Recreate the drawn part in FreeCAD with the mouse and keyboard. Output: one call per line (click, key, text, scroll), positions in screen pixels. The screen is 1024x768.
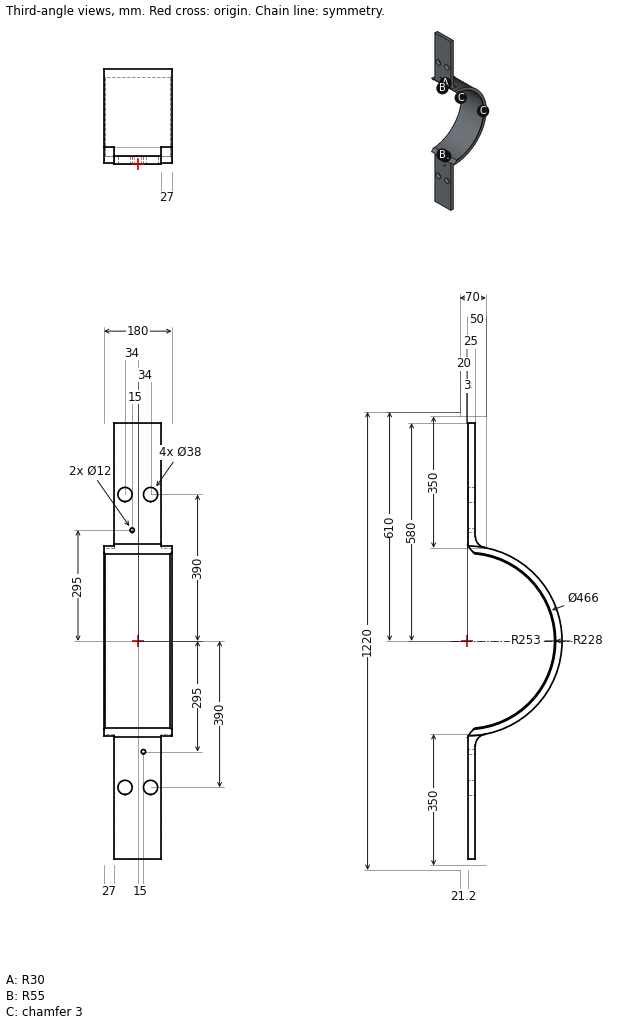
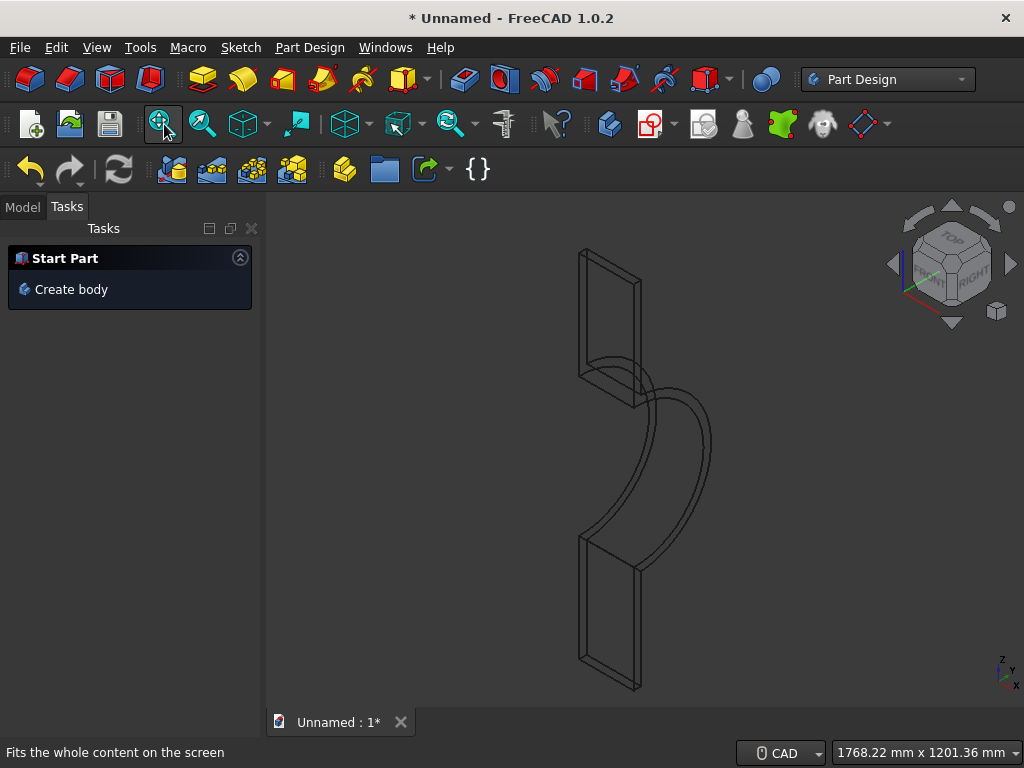
click(614, 378)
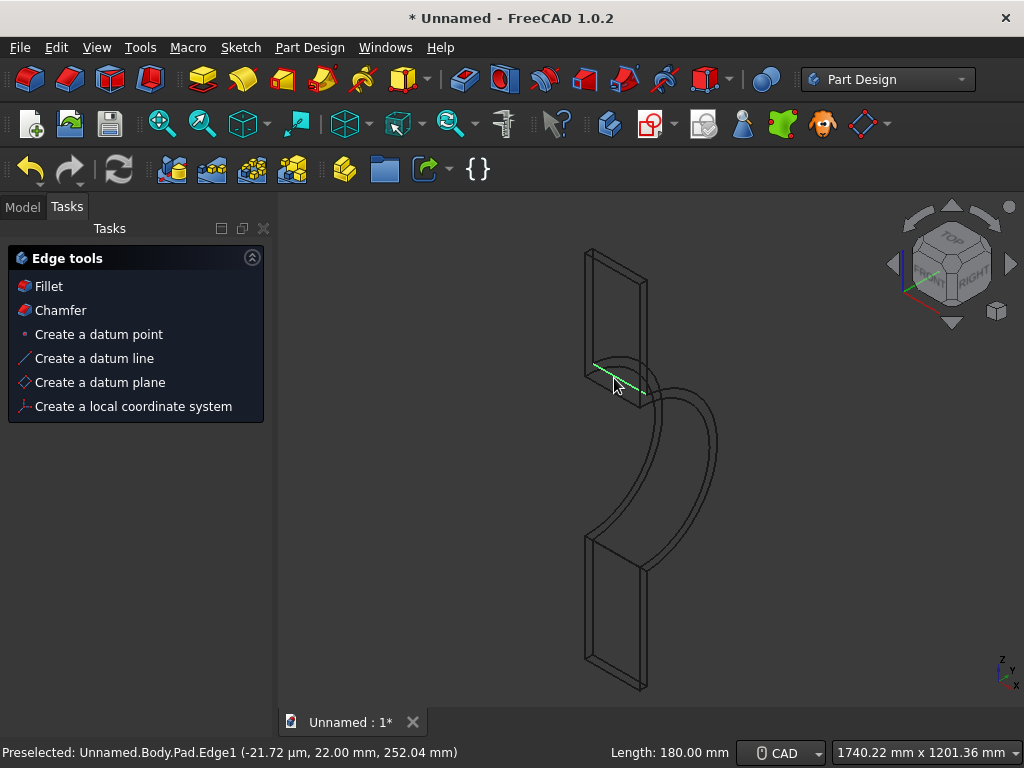
key(2)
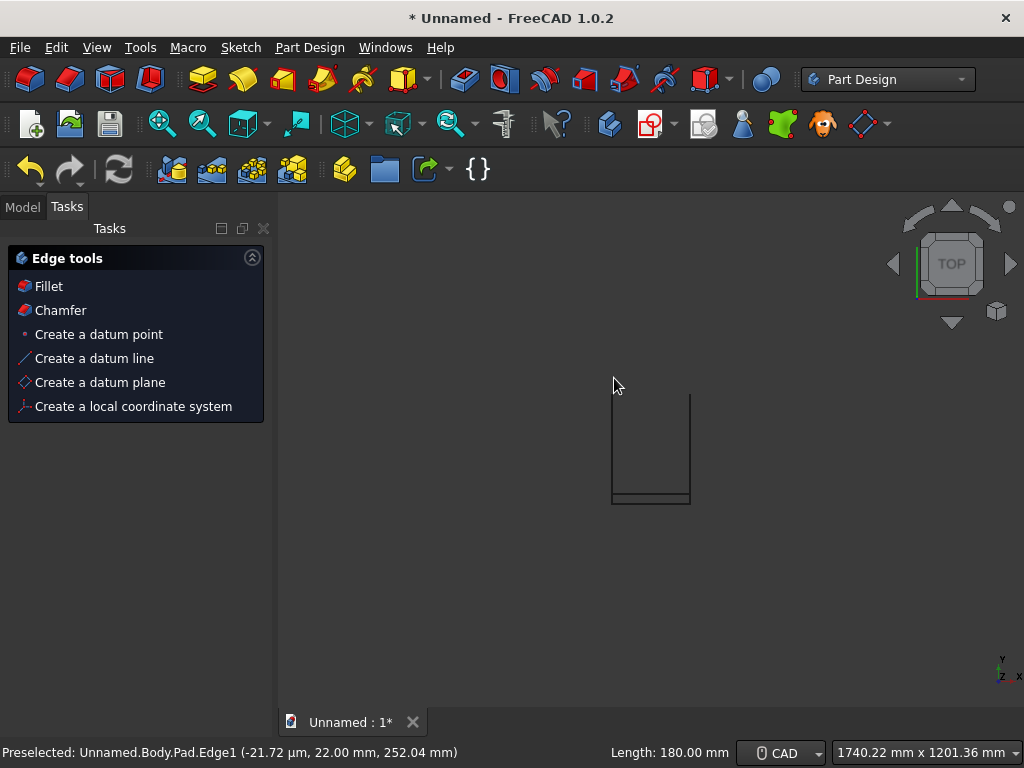
click(164, 124)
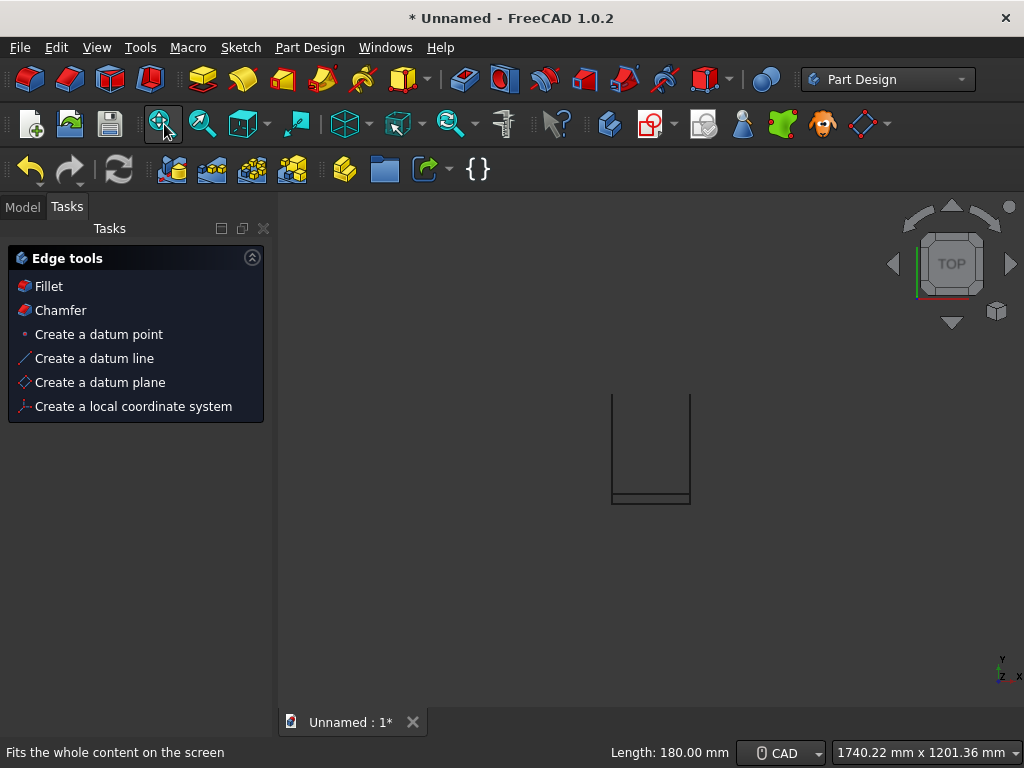
key(1)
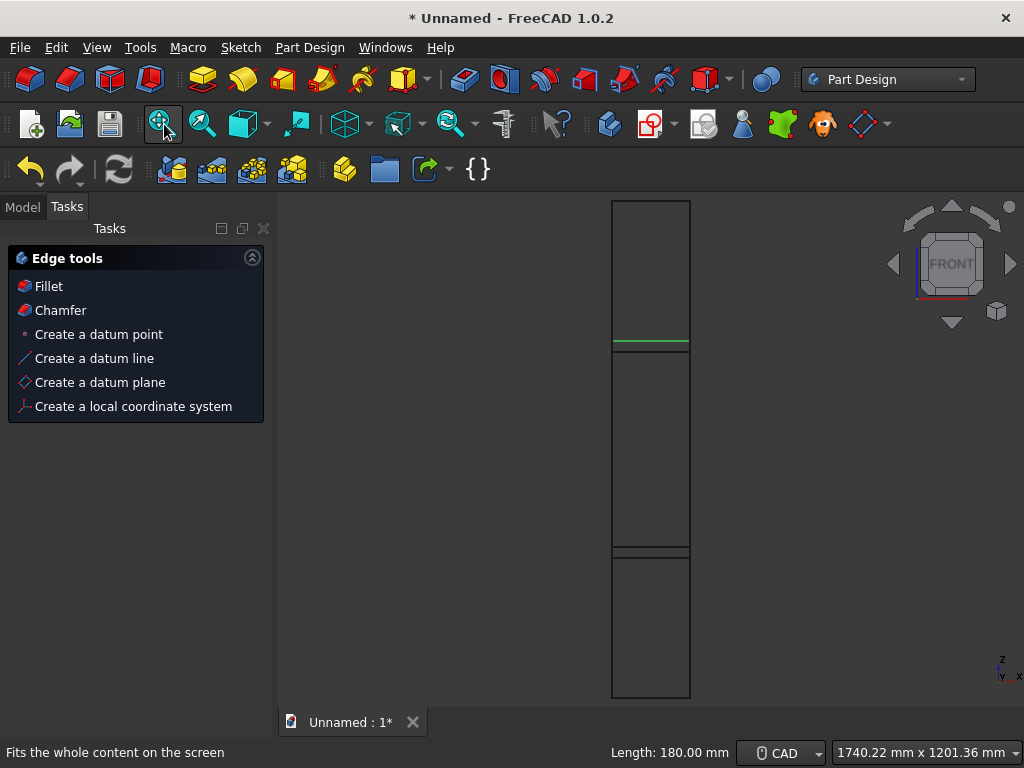
click(651, 557, ctrl)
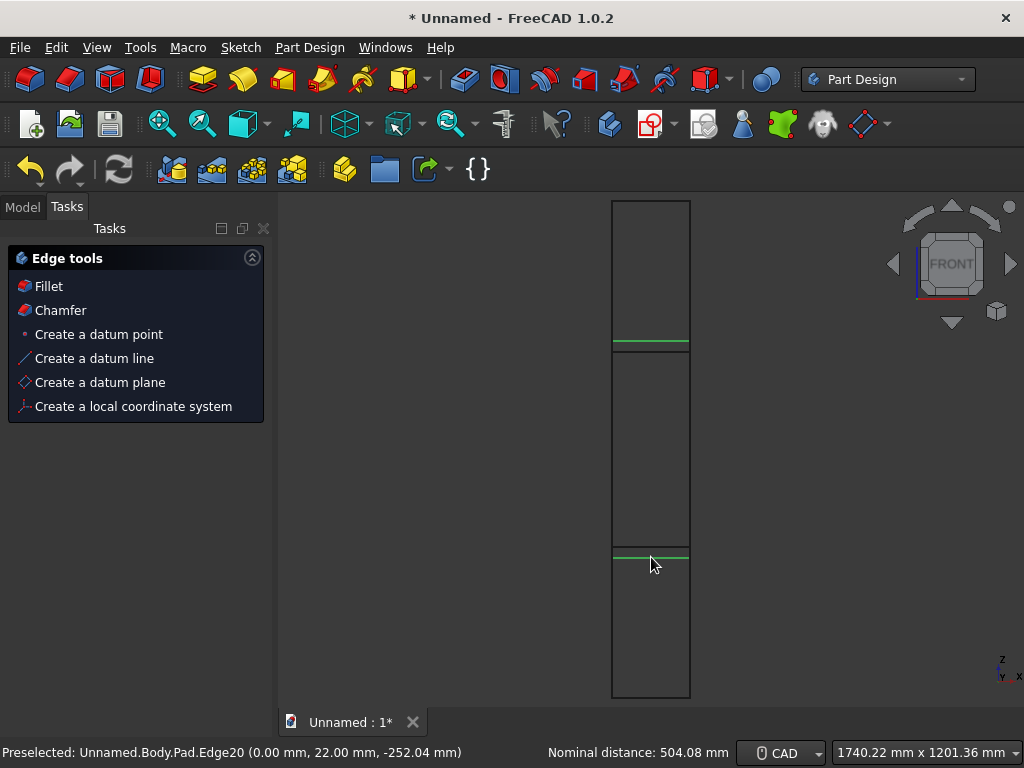
key(v)
key(1)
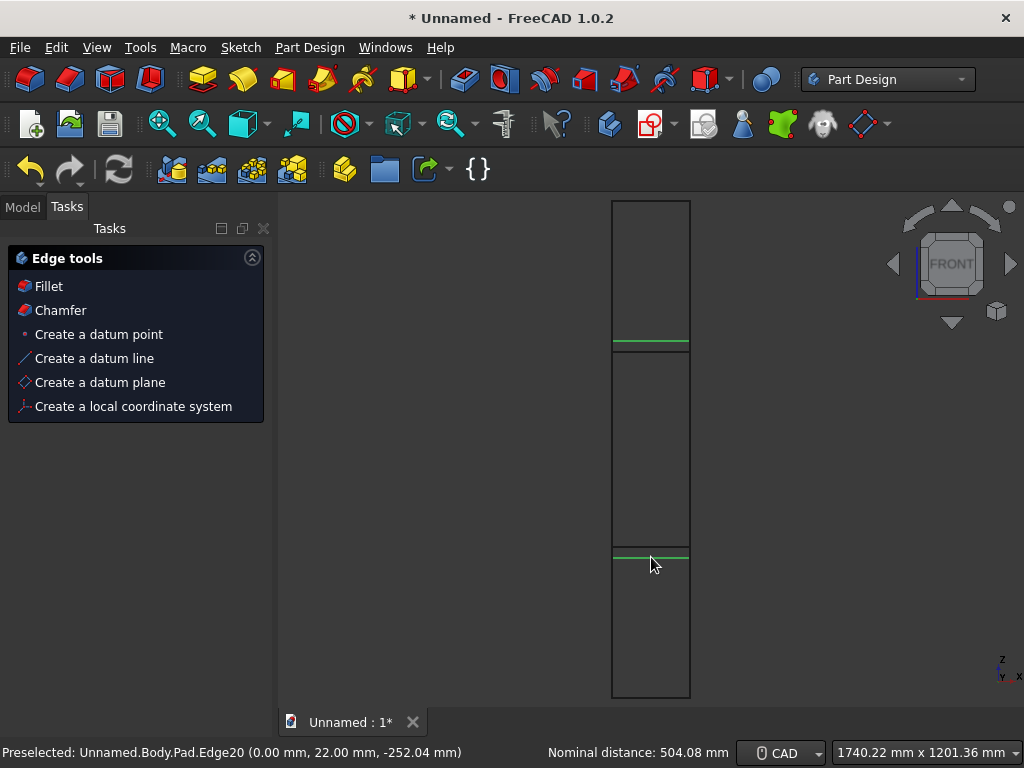
click(30, 80)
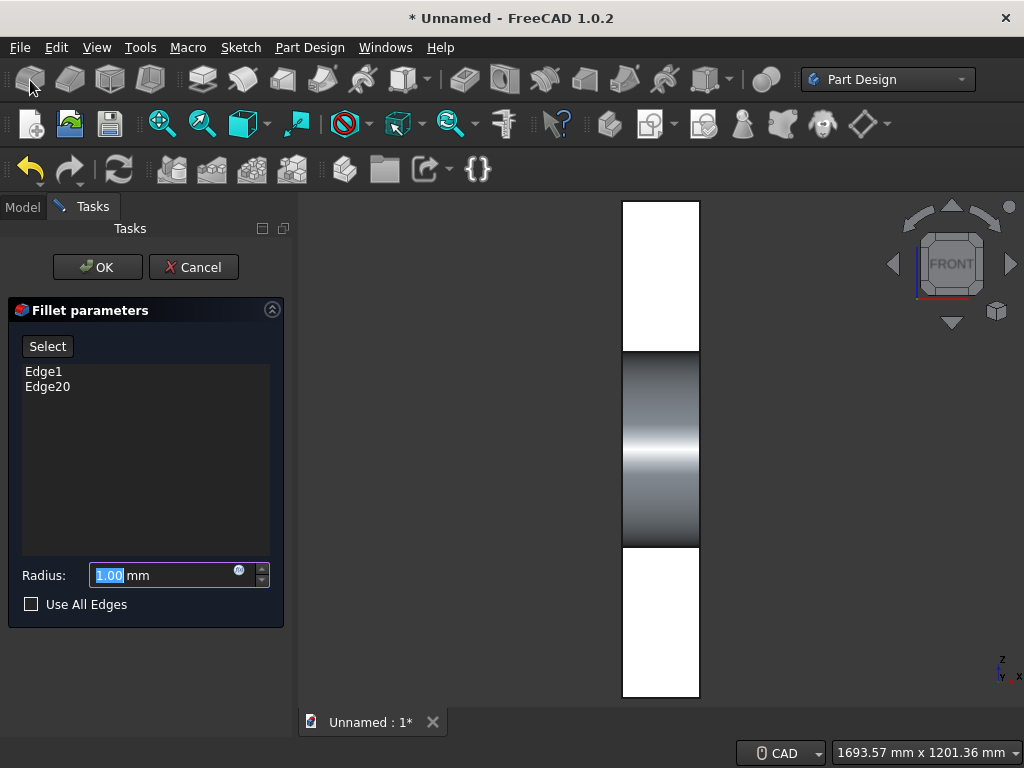
text(30)
key(Tab)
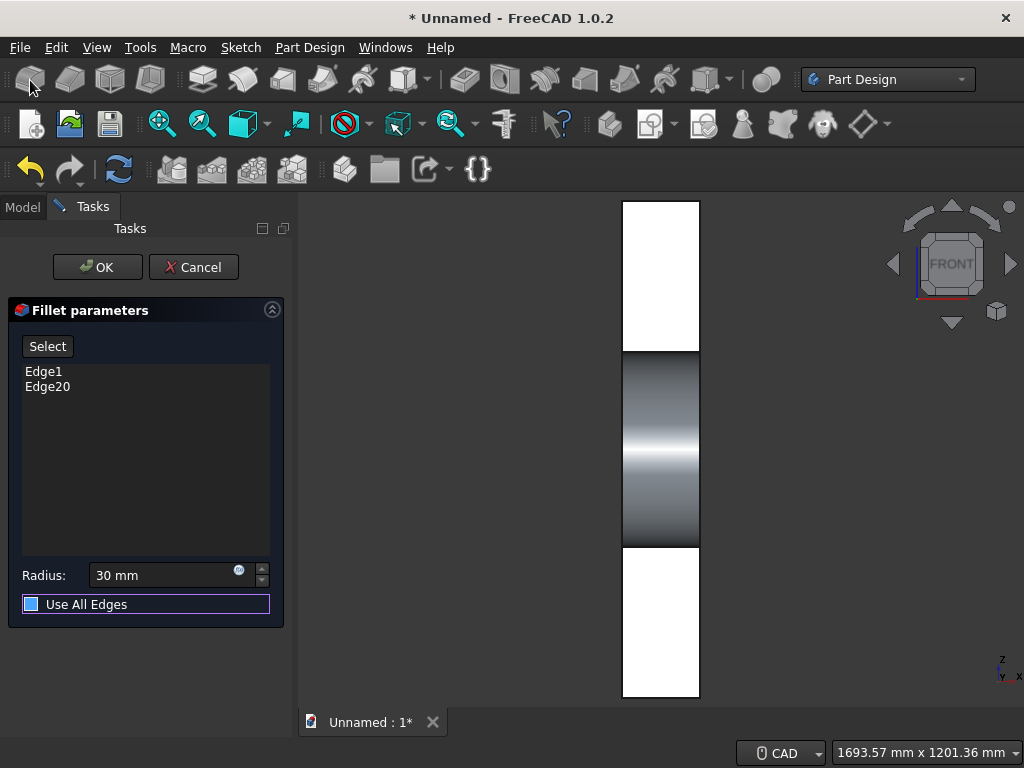
click(98, 267)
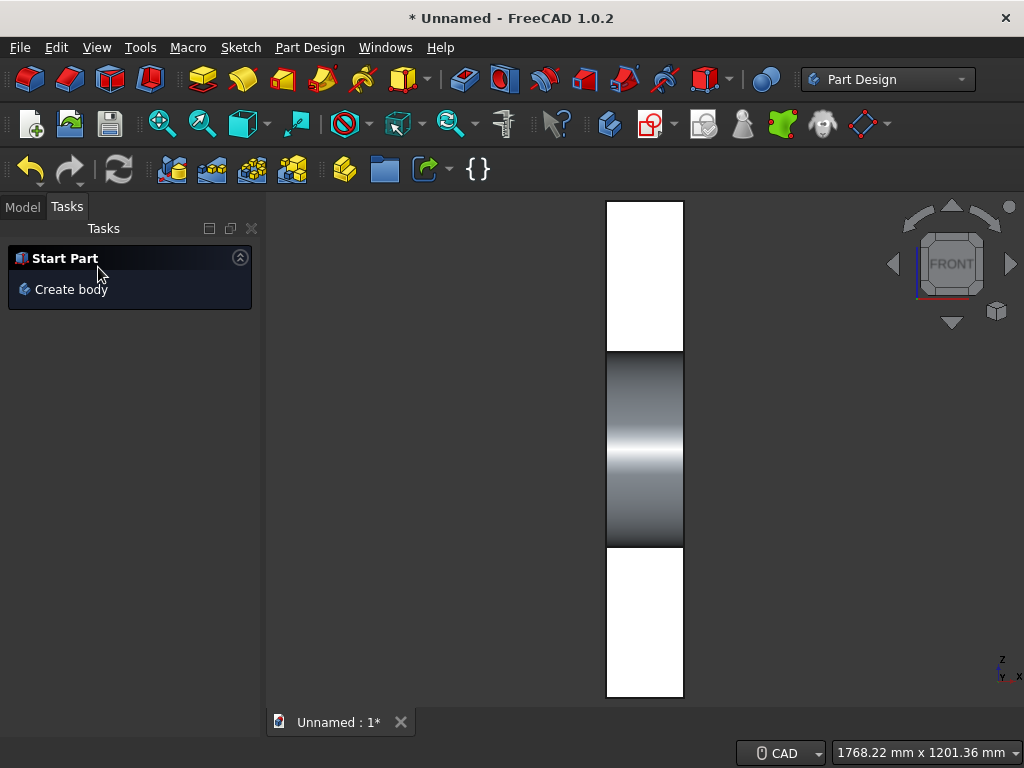
click(645, 546)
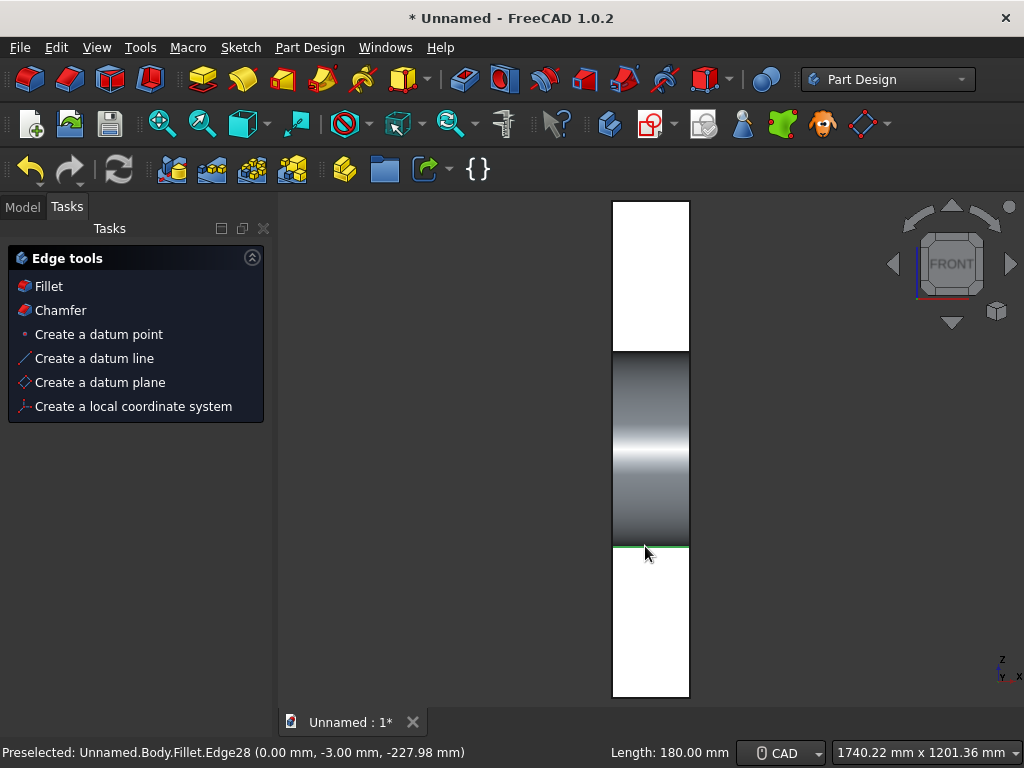
click(651, 351, ctrl)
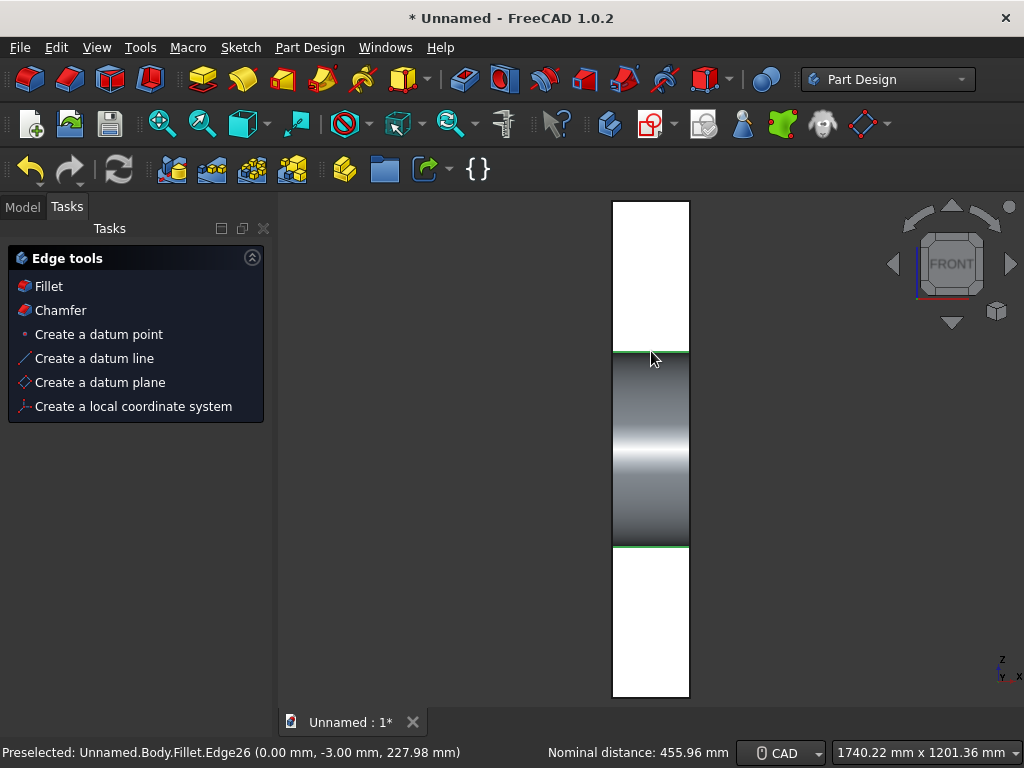
click(30, 80)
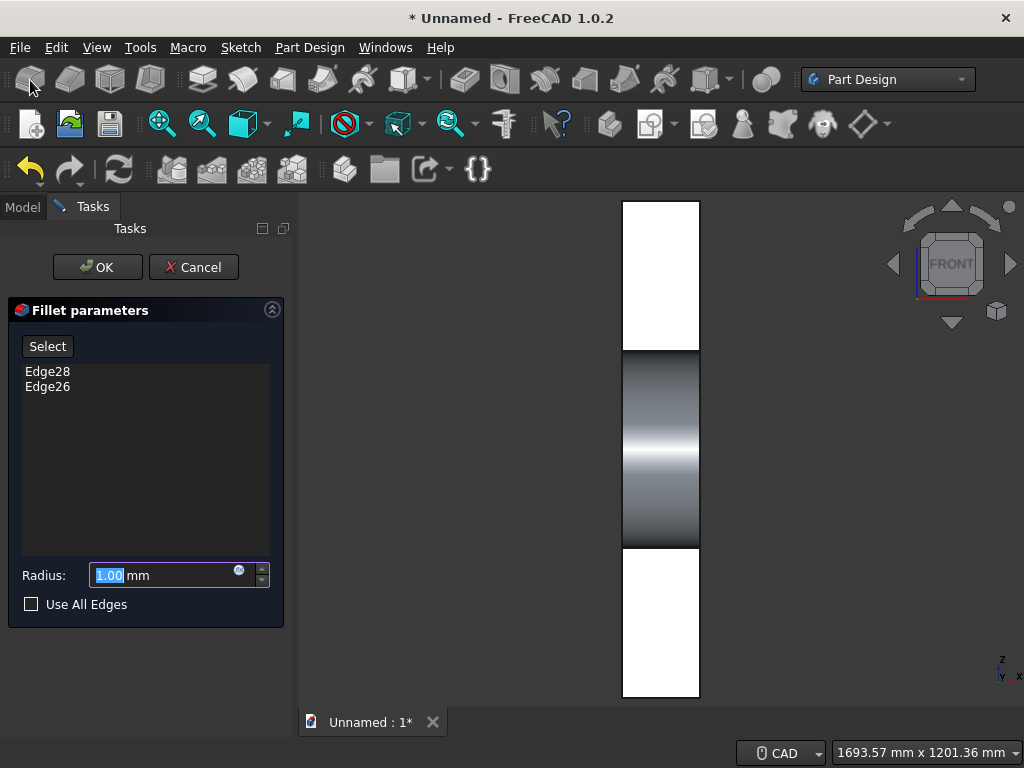
text(55)
key(Tab)